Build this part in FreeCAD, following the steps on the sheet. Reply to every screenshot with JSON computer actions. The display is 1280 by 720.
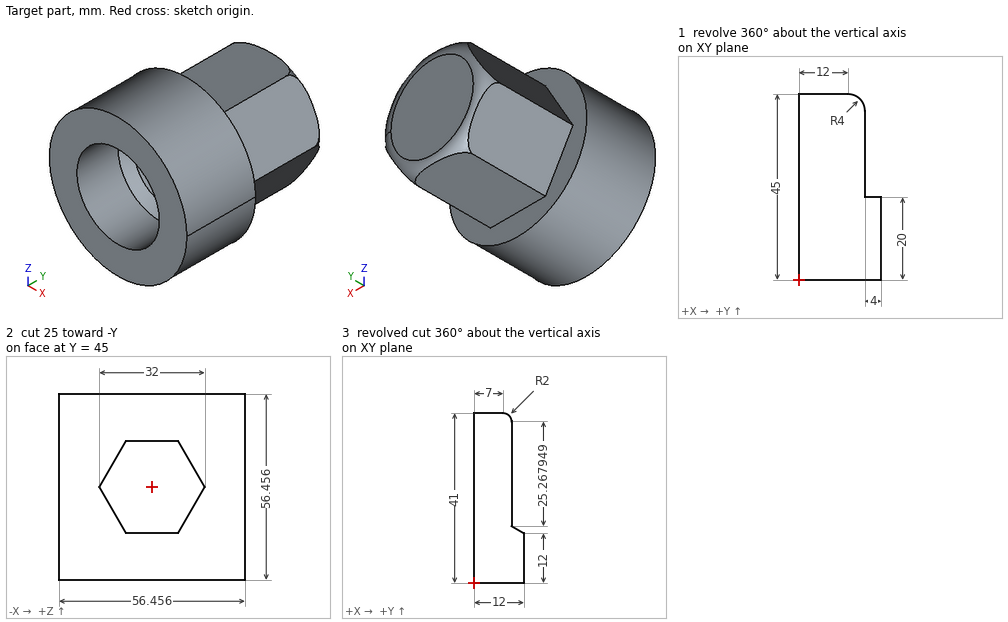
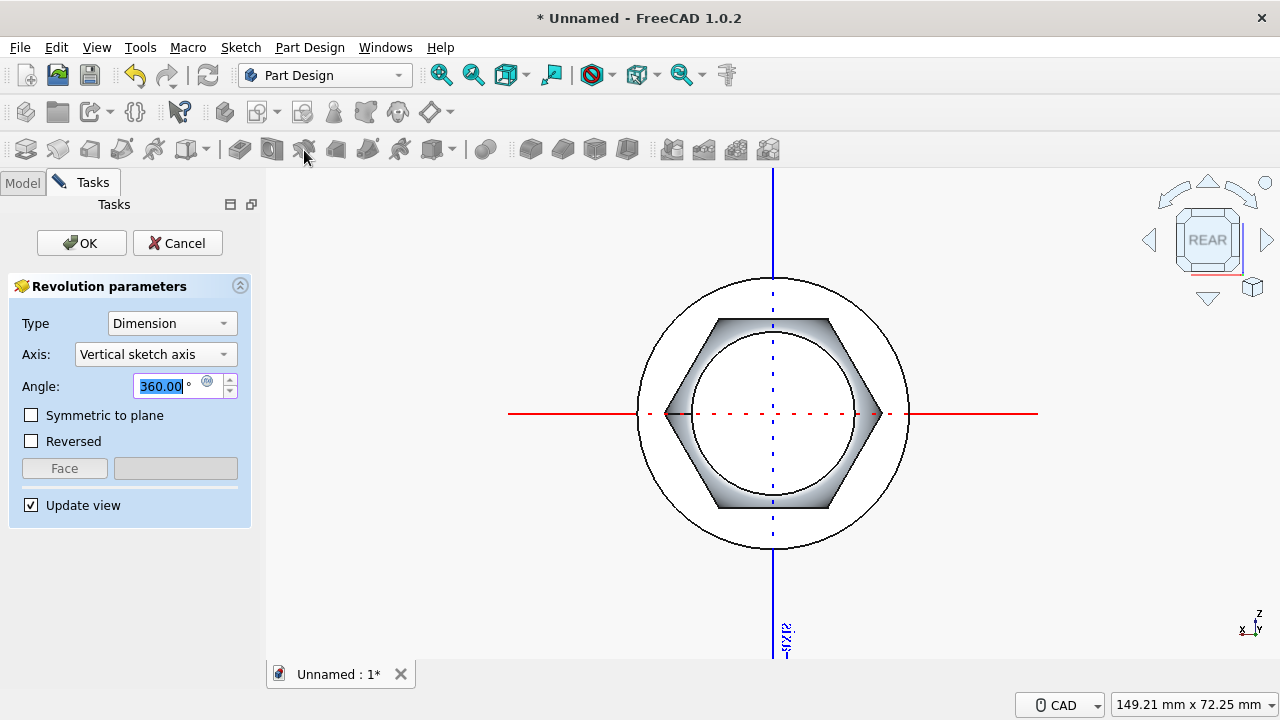
{"action": "left_click", "coordinate": [82, 243]}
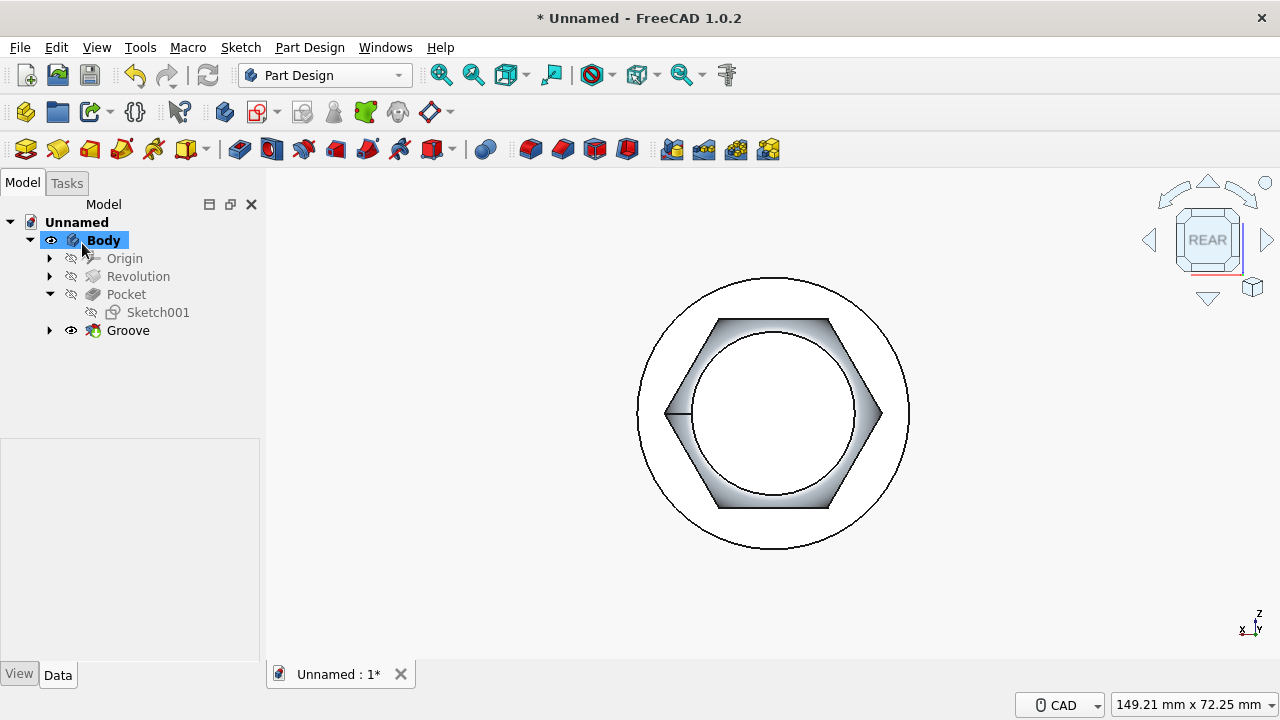
{"action": "key", "text": "0"}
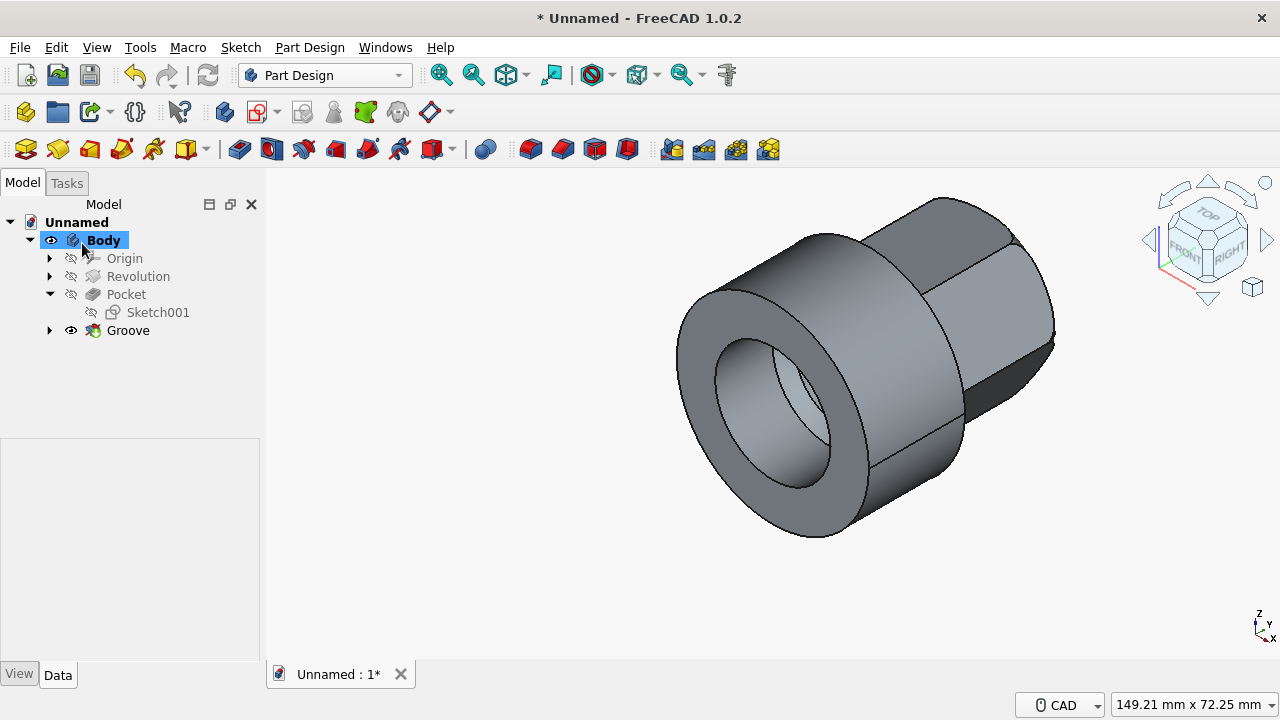
{"action": "key", "text": "v f"}